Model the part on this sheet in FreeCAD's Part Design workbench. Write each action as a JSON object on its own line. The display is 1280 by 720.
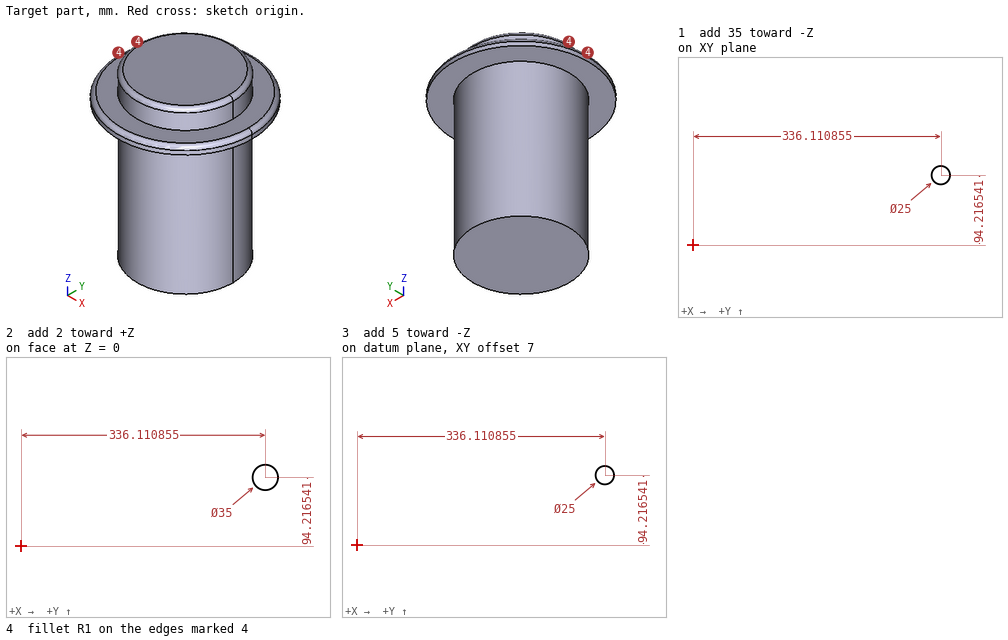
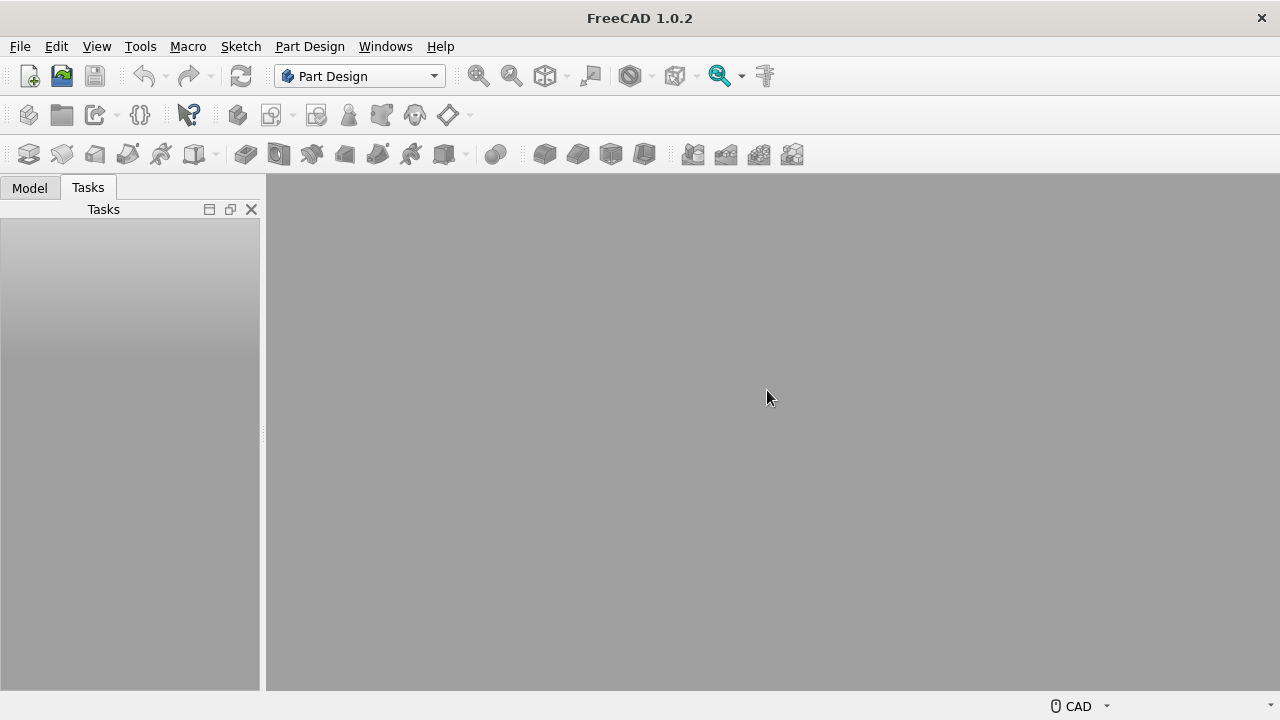
{"action": "left_click", "coordinate": [29, 76]}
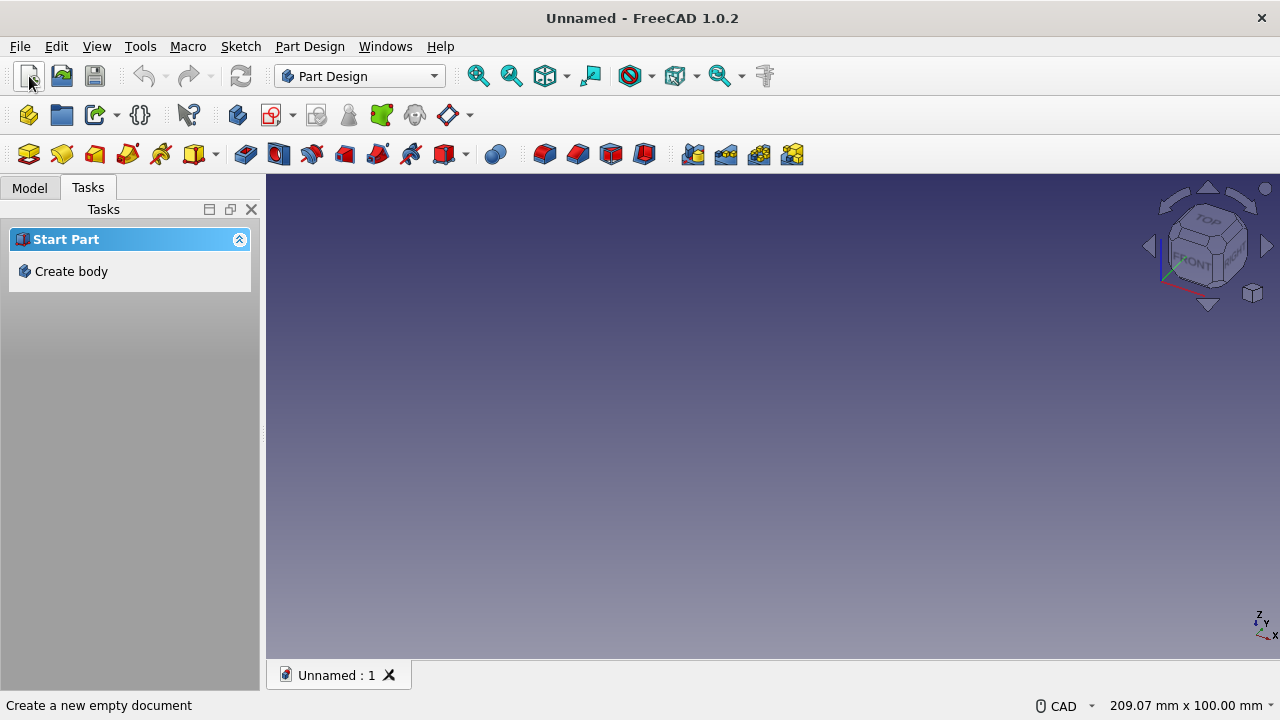
{"action": "left_click", "coordinate": [270, 116]}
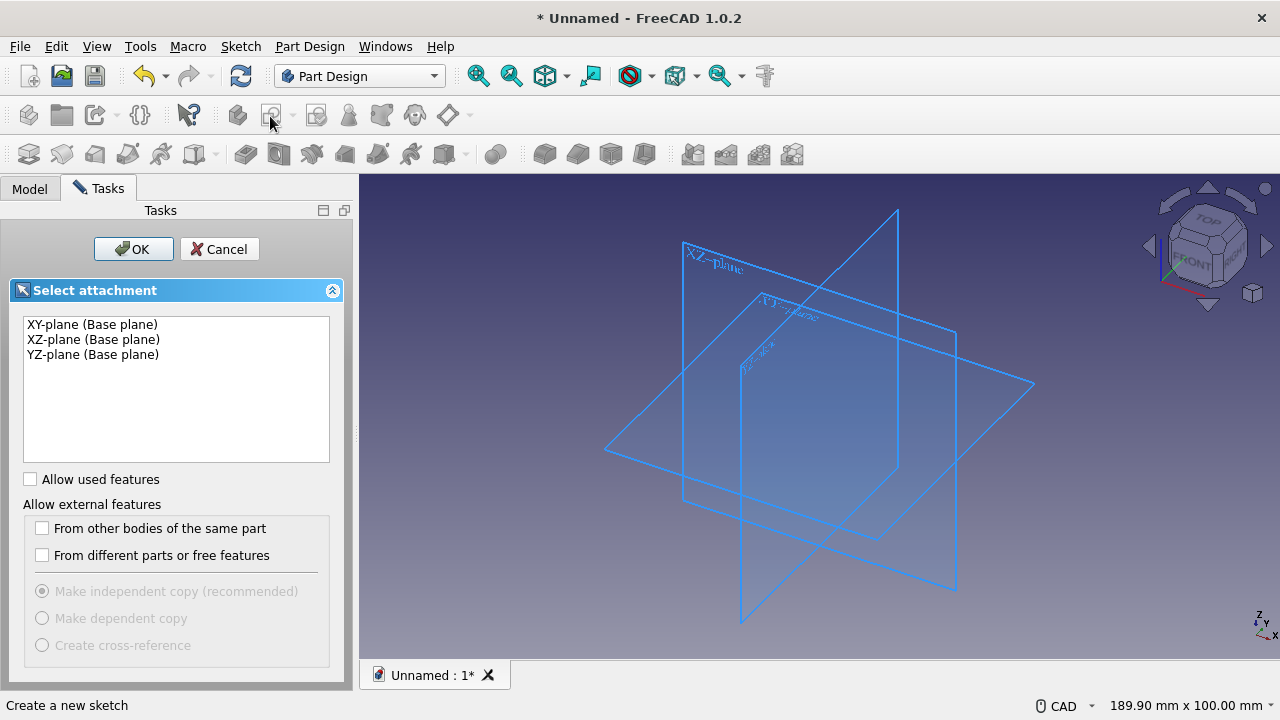
{"action": "left_click", "coordinate": [84, 324]}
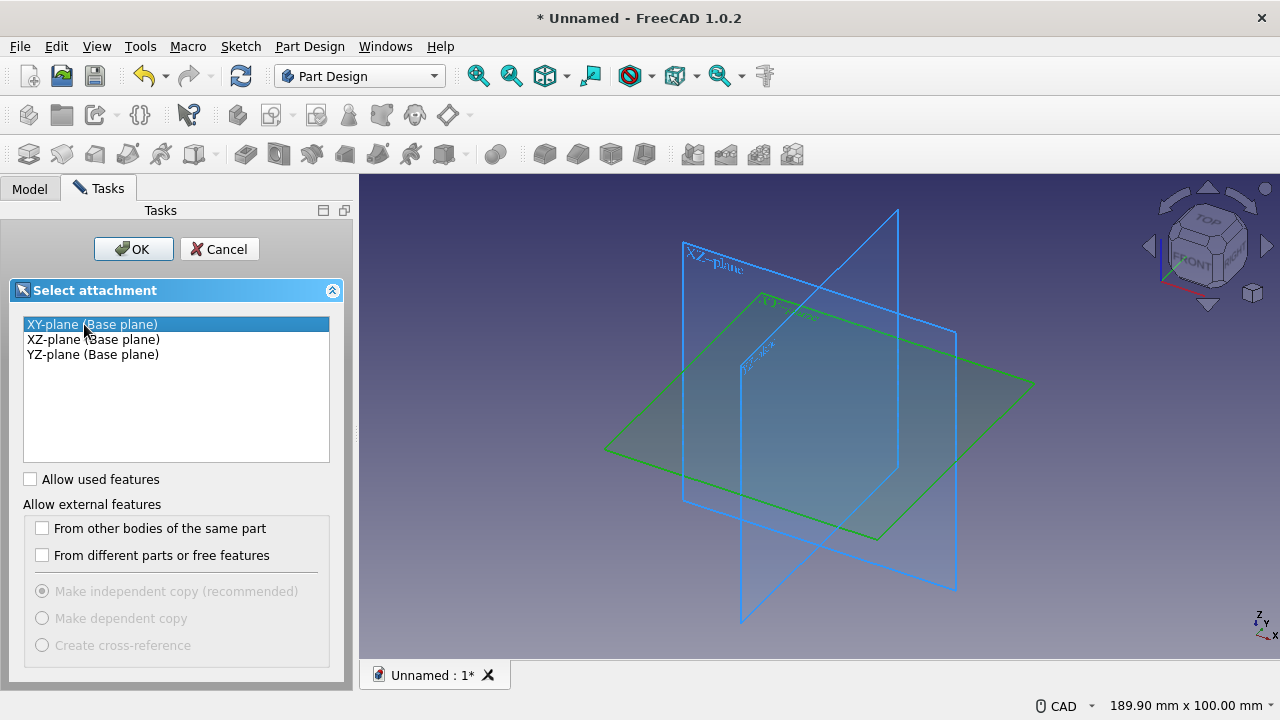
{"action": "left_click", "coordinate": [134, 249]}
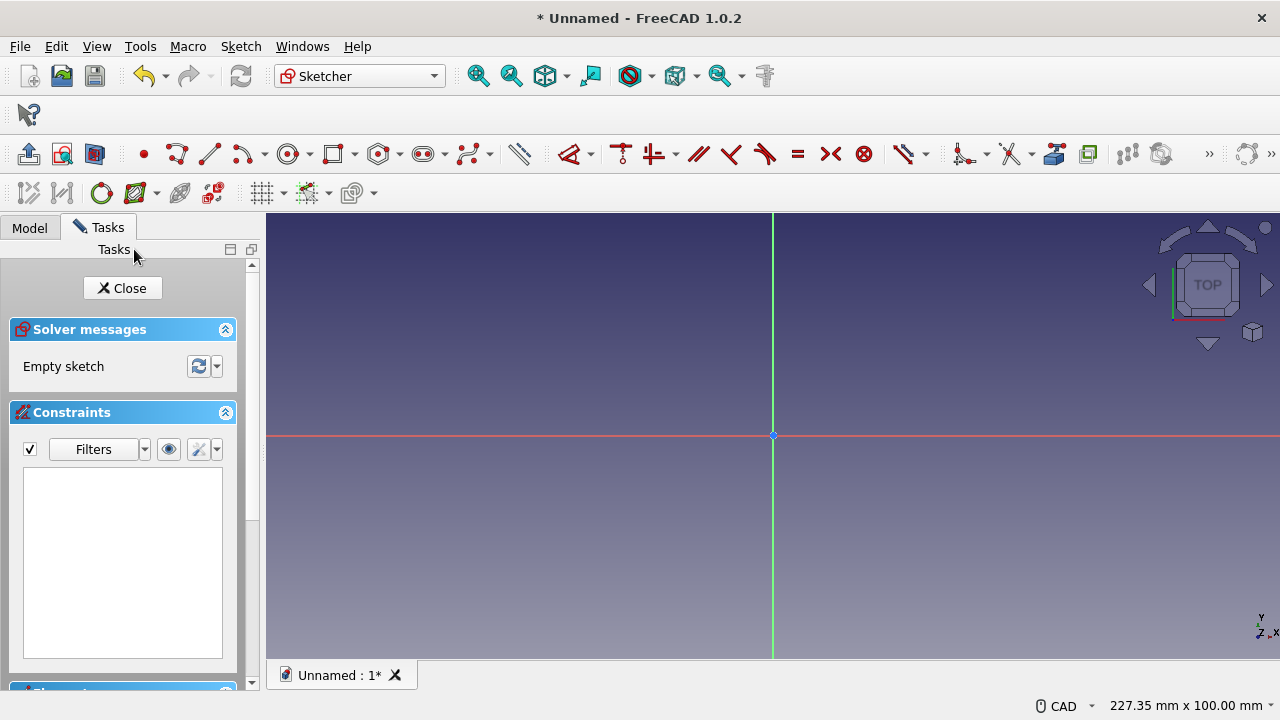
{"action": "scroll", "coordinate": [704, 436], "scroll_direction": "down", "scroll_amount": 5}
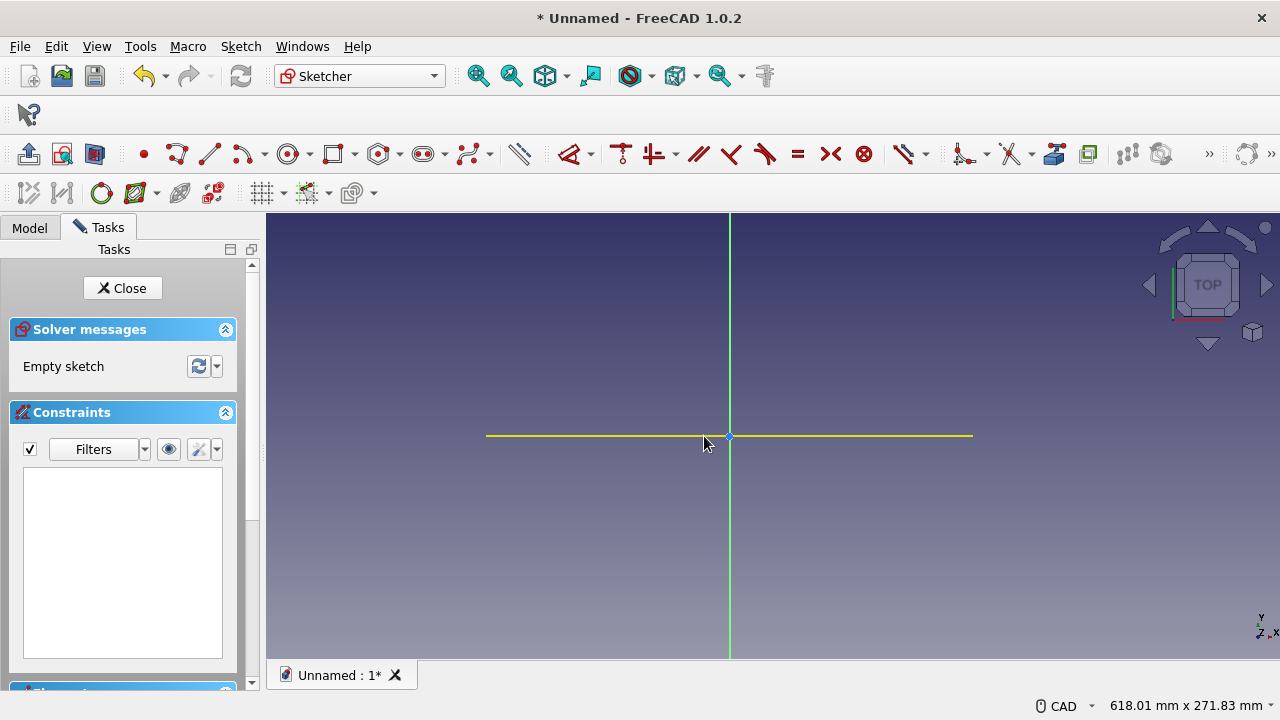
{"action": "scroll", "coordinate": [704, 436], "scroll_direction": "down", "scroll_amount": 5}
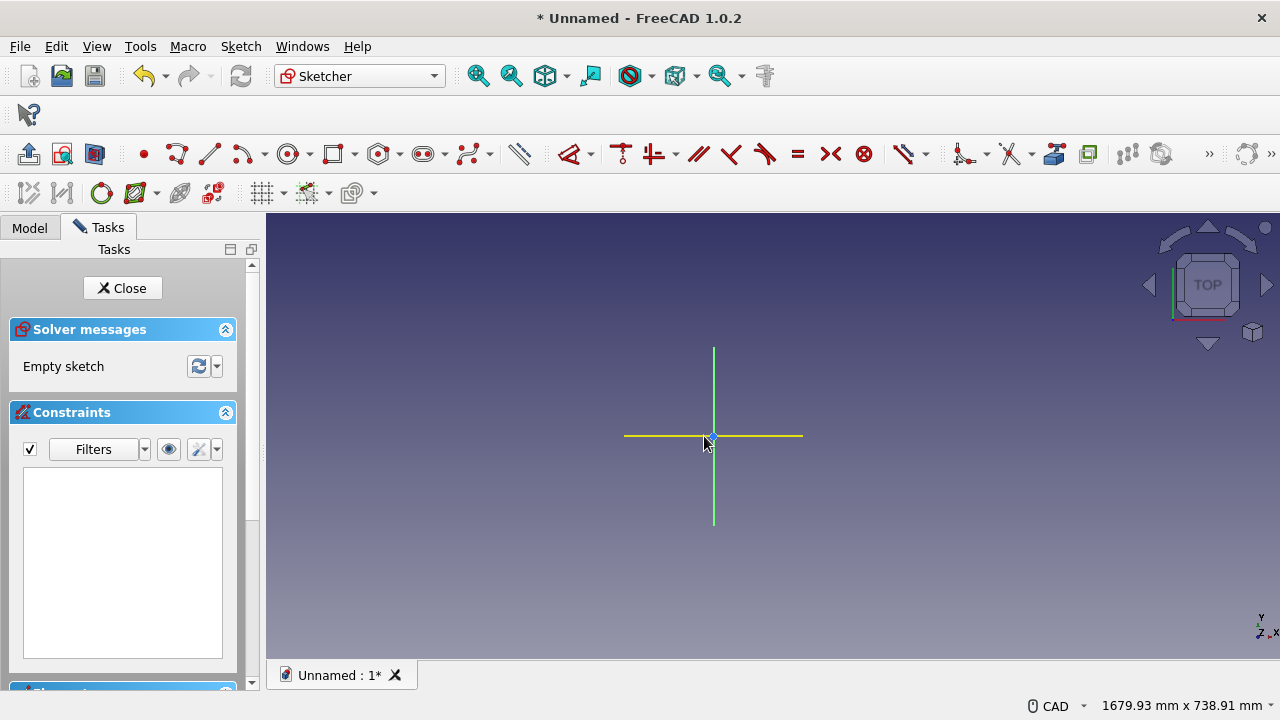
{"action": "scroll", "coordinate": [928, 377], "scroll_direction": "up", "scroll_amount": 15}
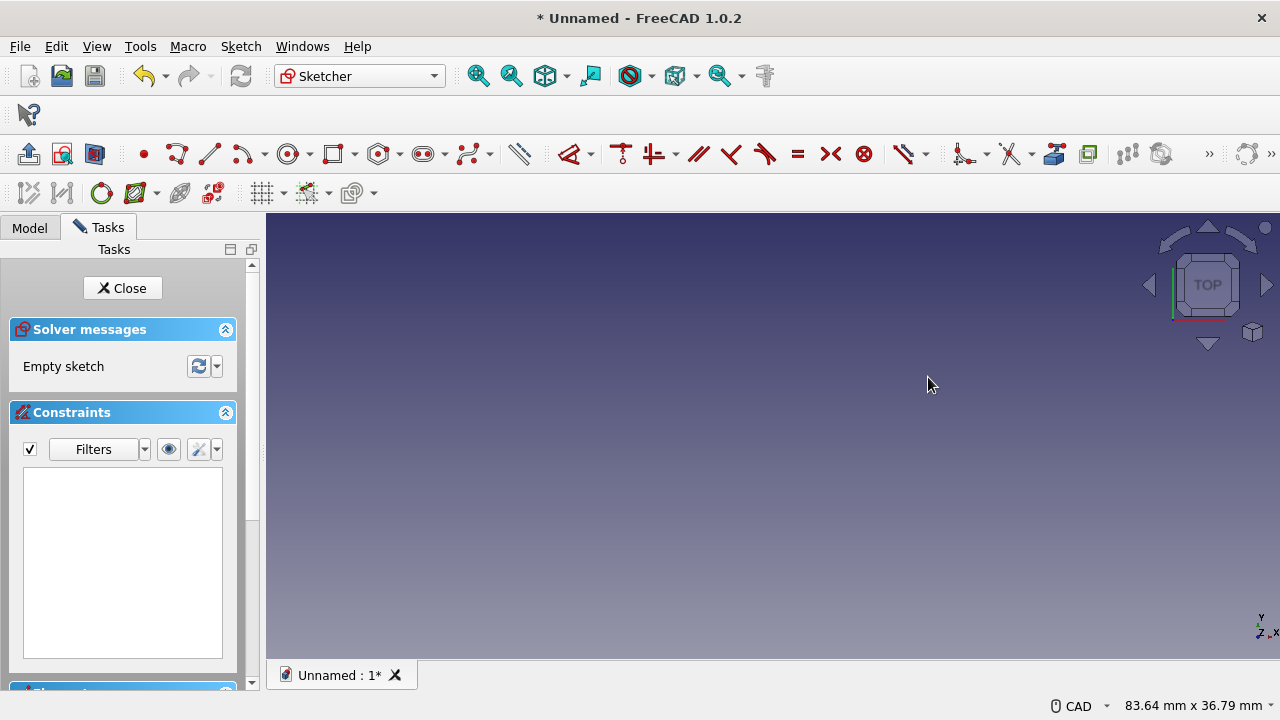
{"action": "left_click", "coordinate": [288, 154]}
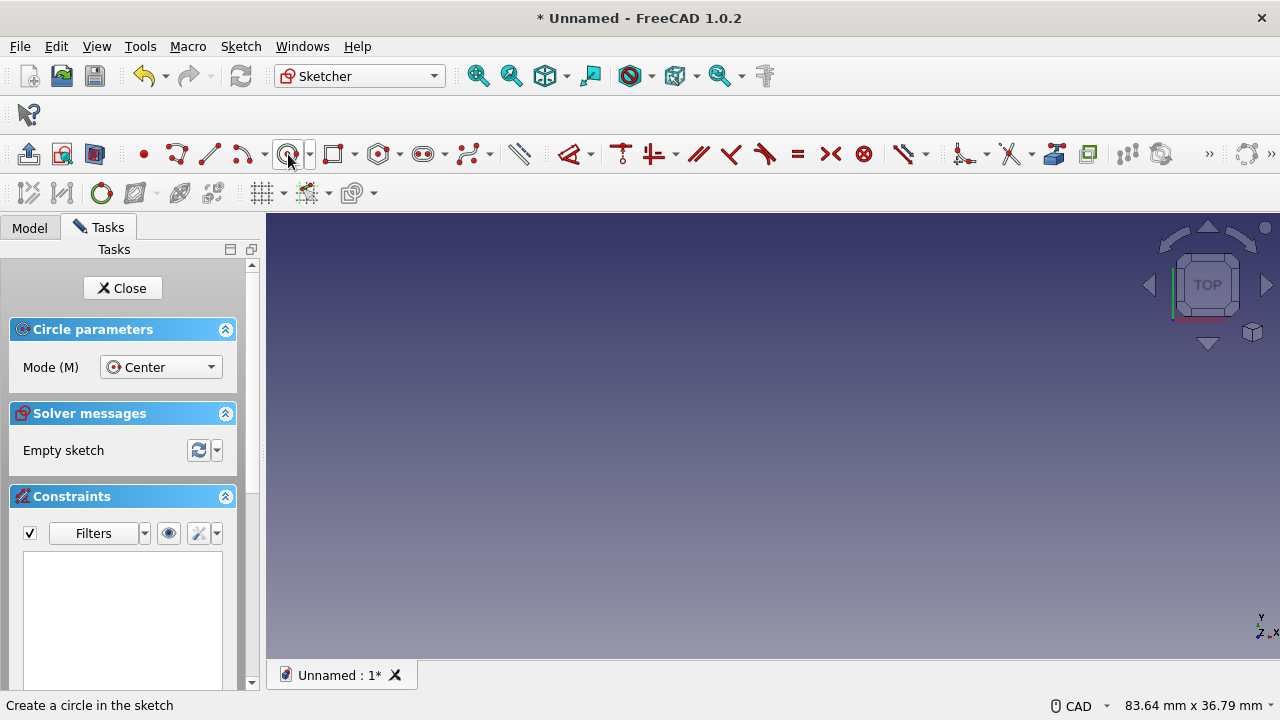
{"action": "left_click", "coordinate": [686, 421]}
{"action": "mouse_move", "coordinate": [793, 314]}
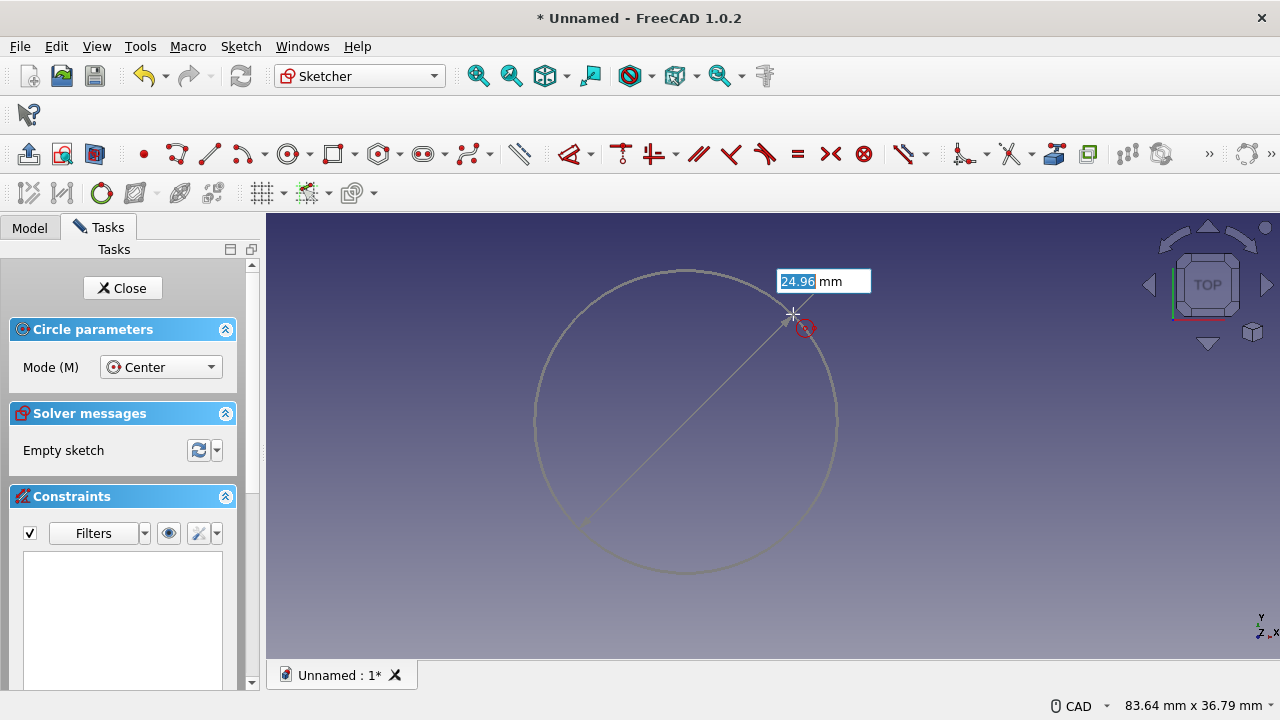
{"action": "type", "text": "25"}
{"action": "key", "text": "Return"}
{"action": "key", "text": "Escape"}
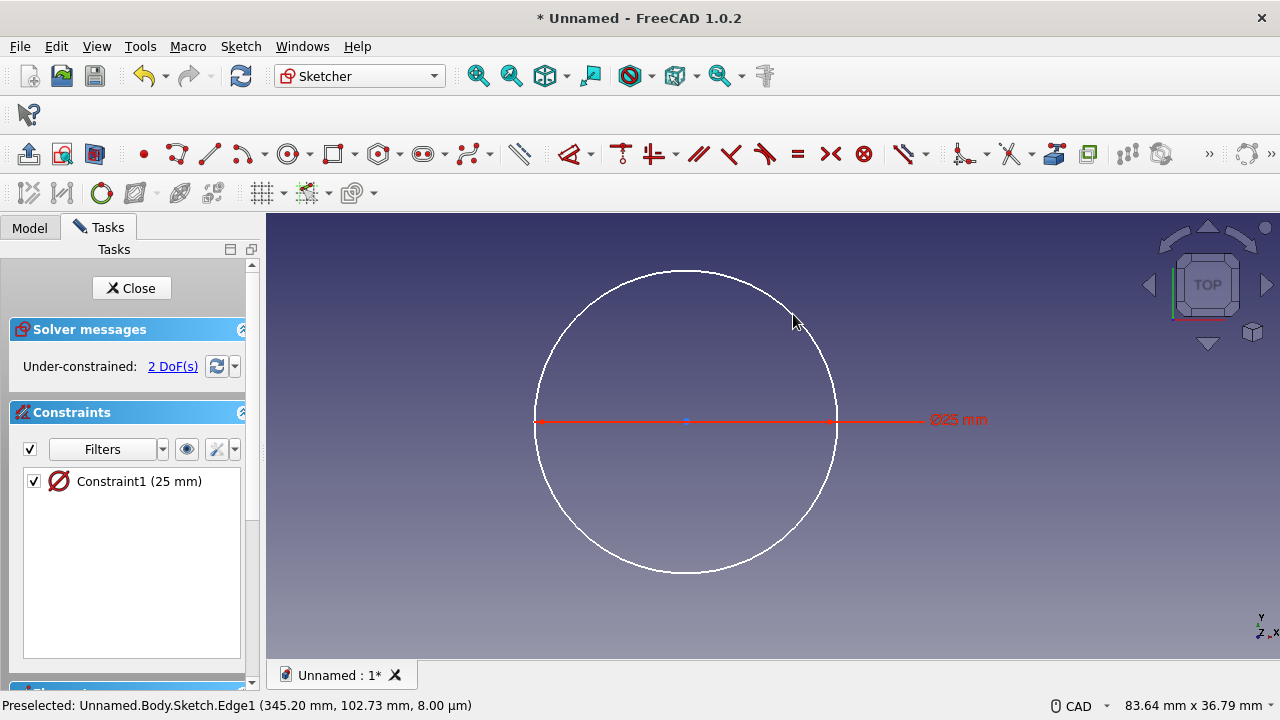
{"action": "left_click", "coordinate": [568, 154]}